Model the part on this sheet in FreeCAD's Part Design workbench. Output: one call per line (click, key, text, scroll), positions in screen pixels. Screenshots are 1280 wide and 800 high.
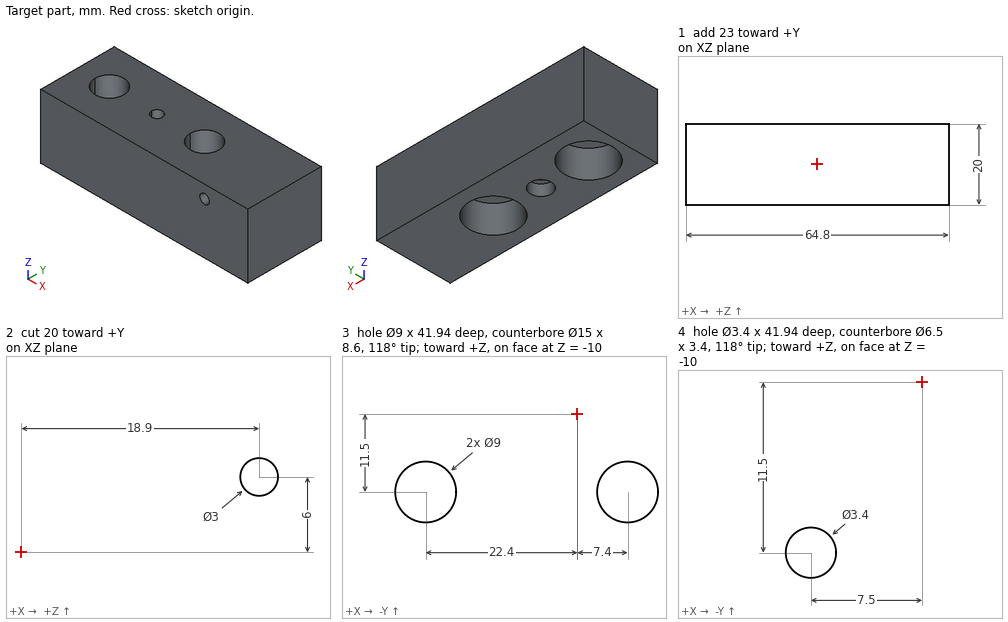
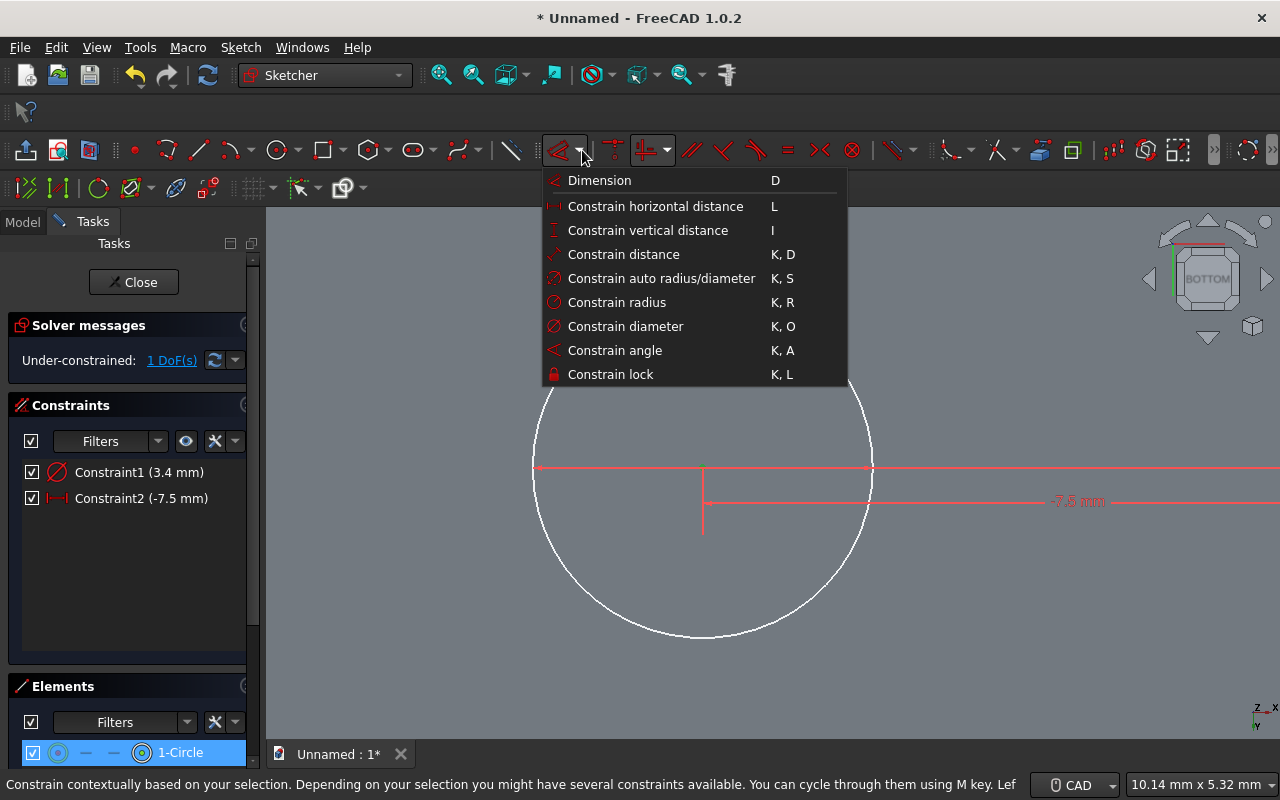
click(695, 230)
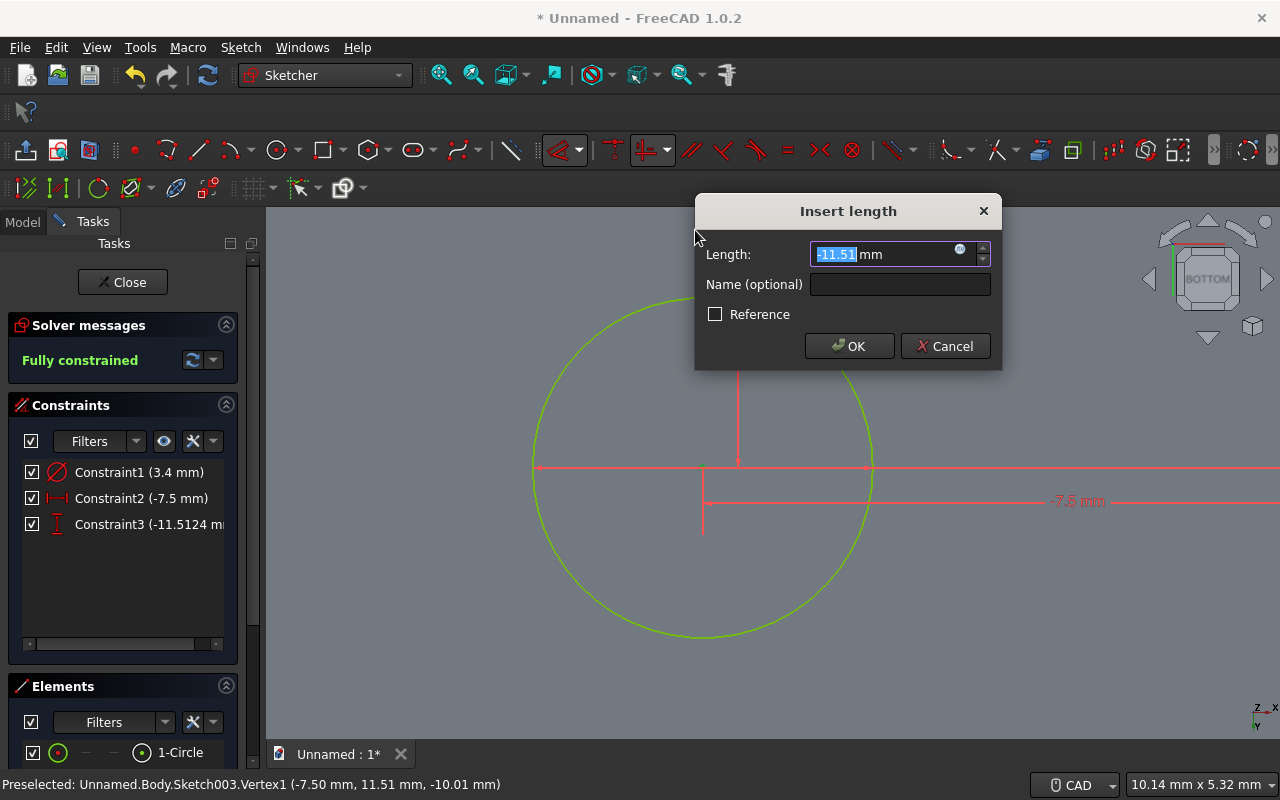
text(-11.5)
key(Return)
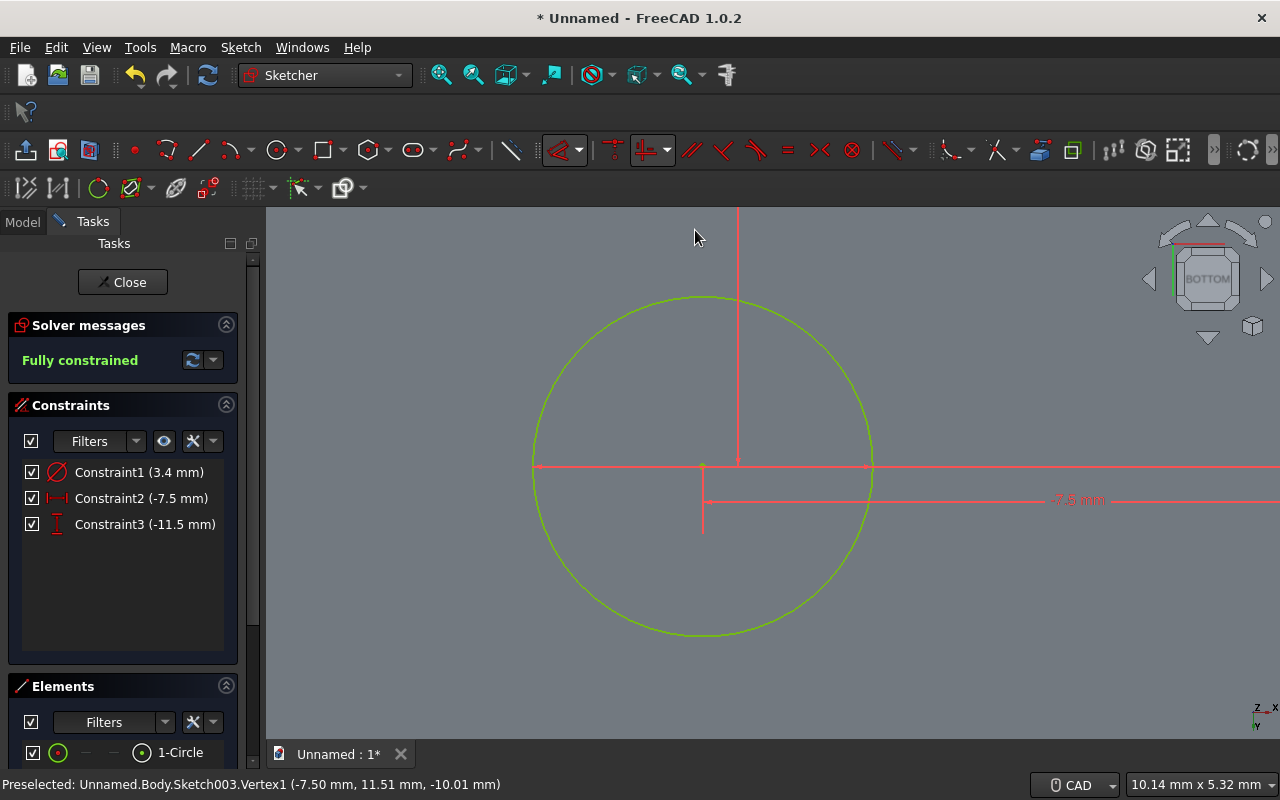
click(123, 282)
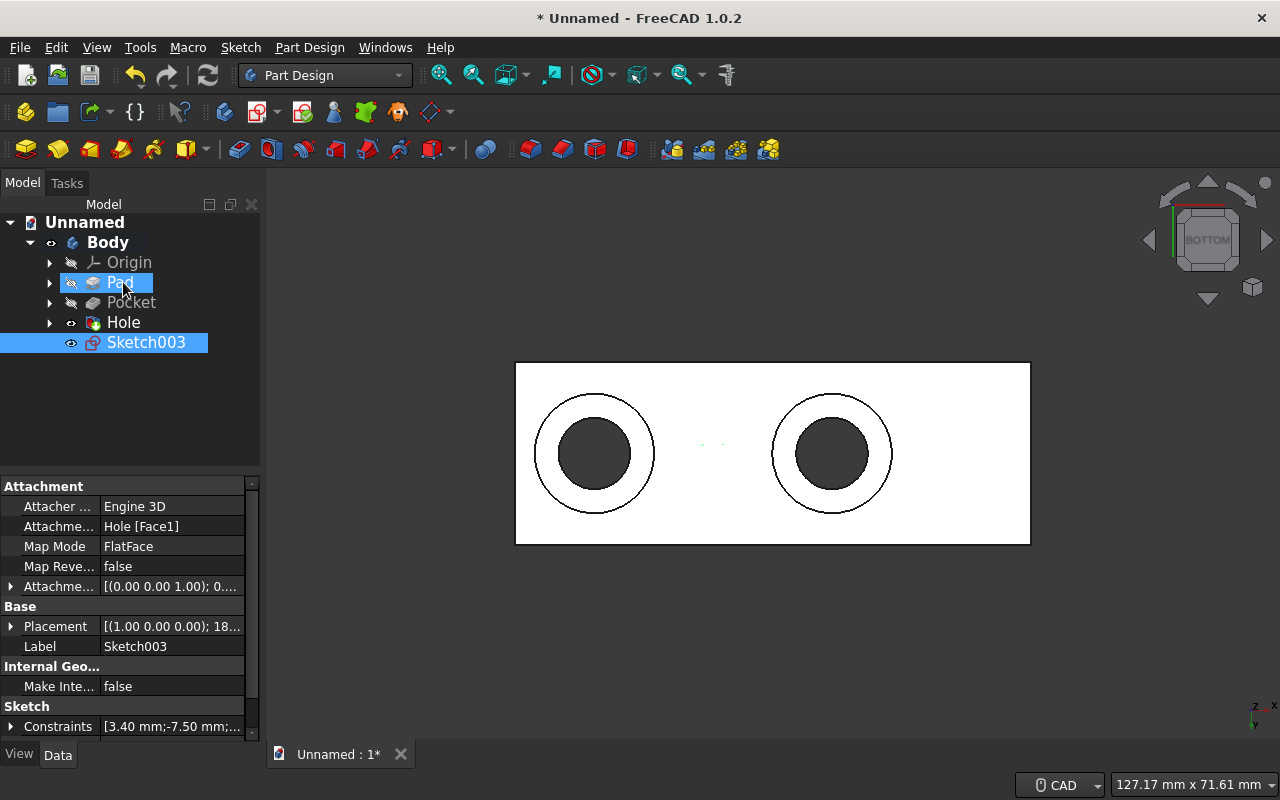
click(272, 150)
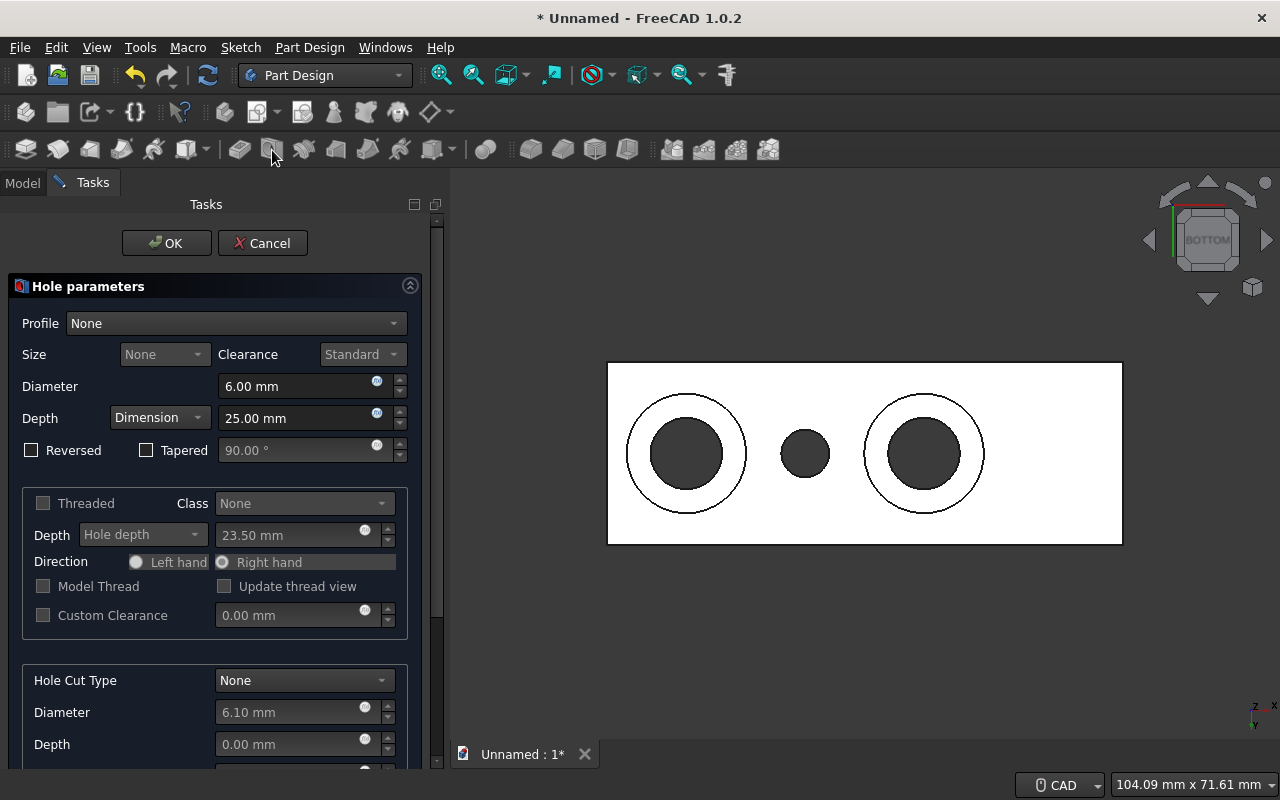
triple_click(305, 386)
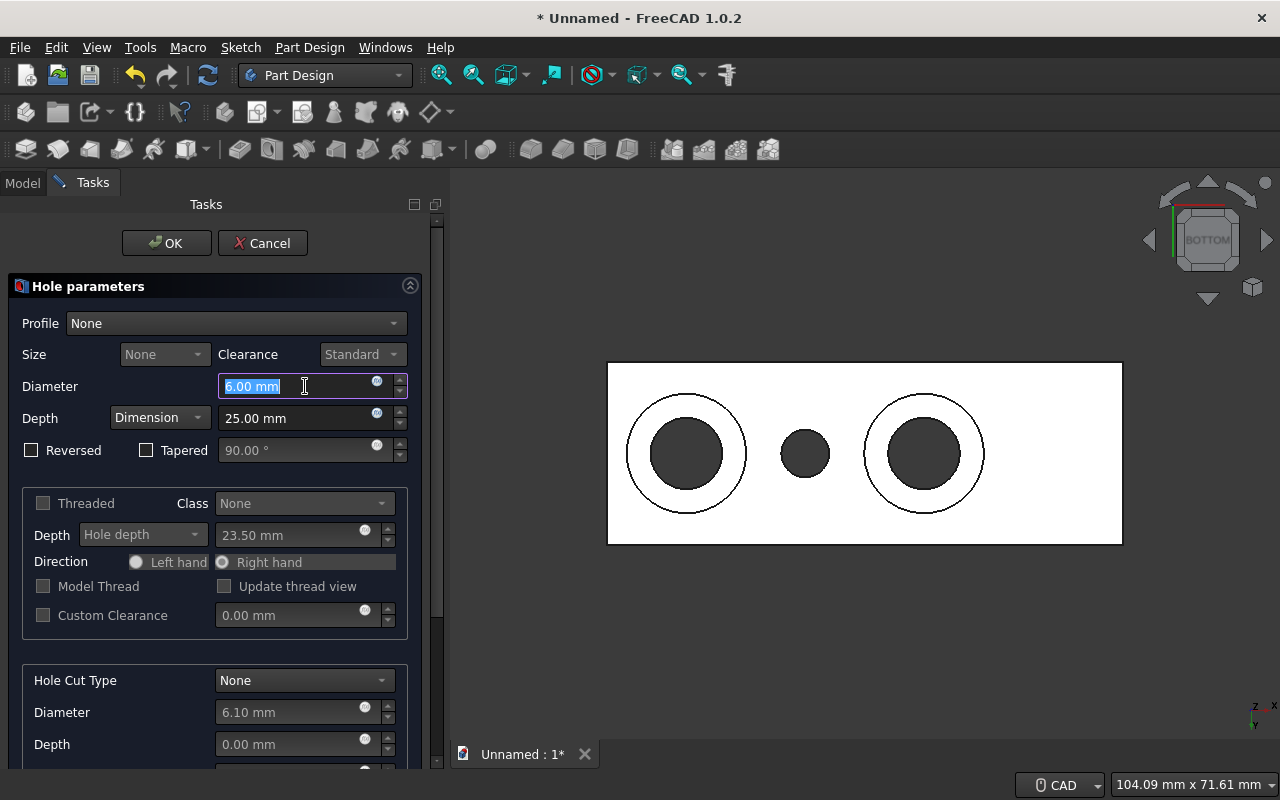
text(3.4)
key(Tab)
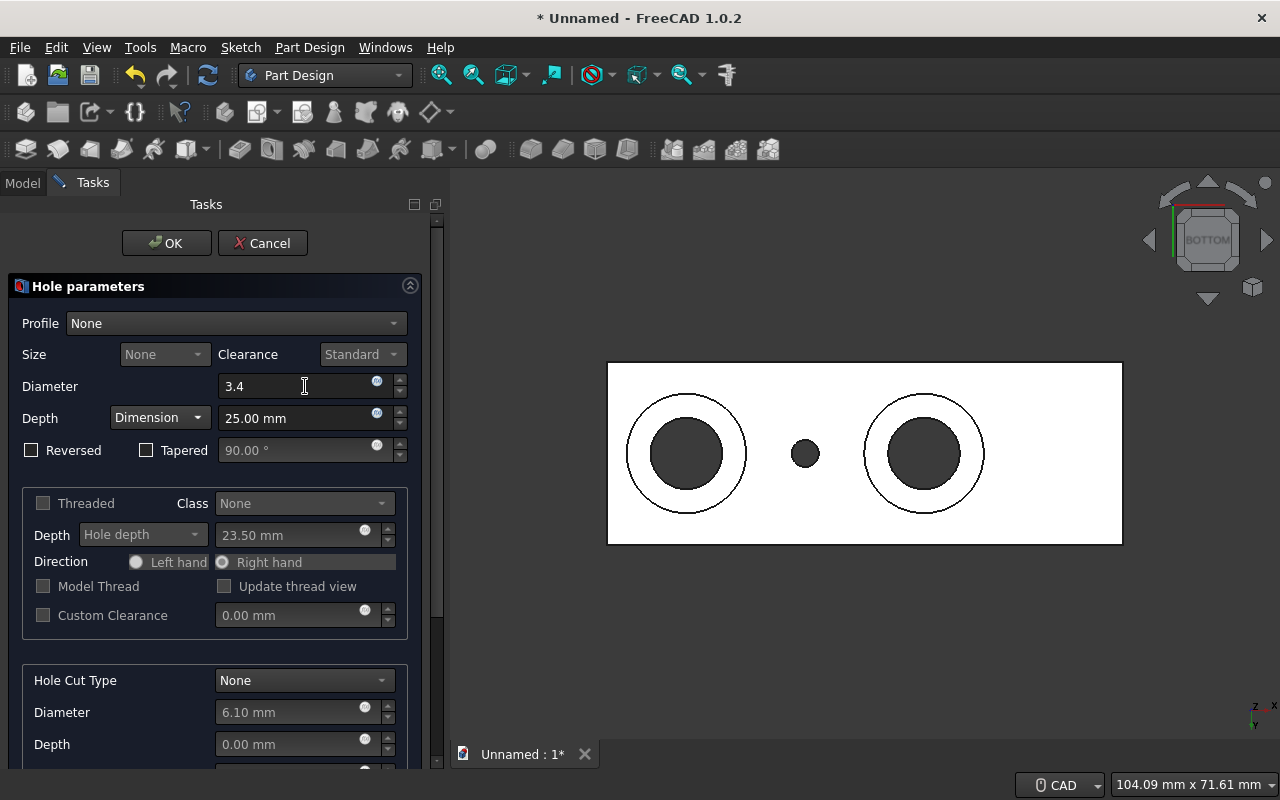
triple_click(305, 418)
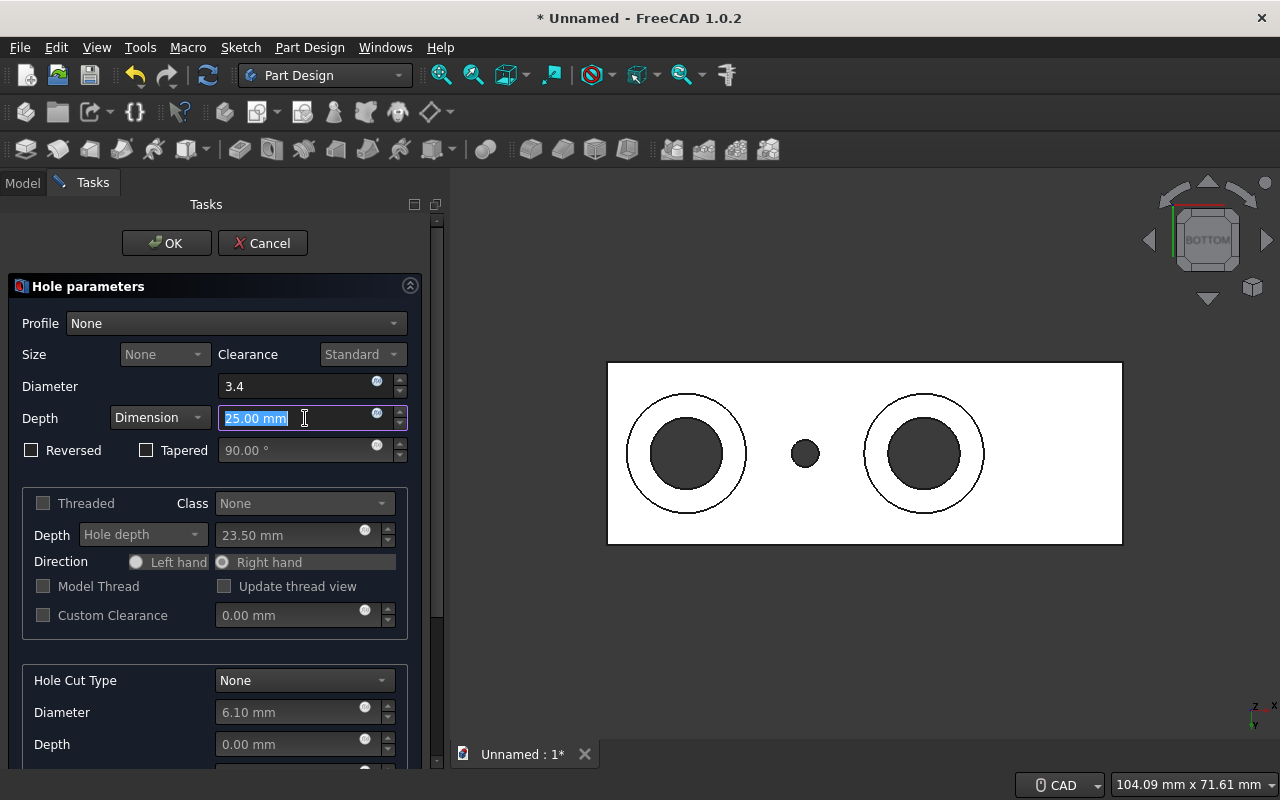
text(41.94)
key(Tab)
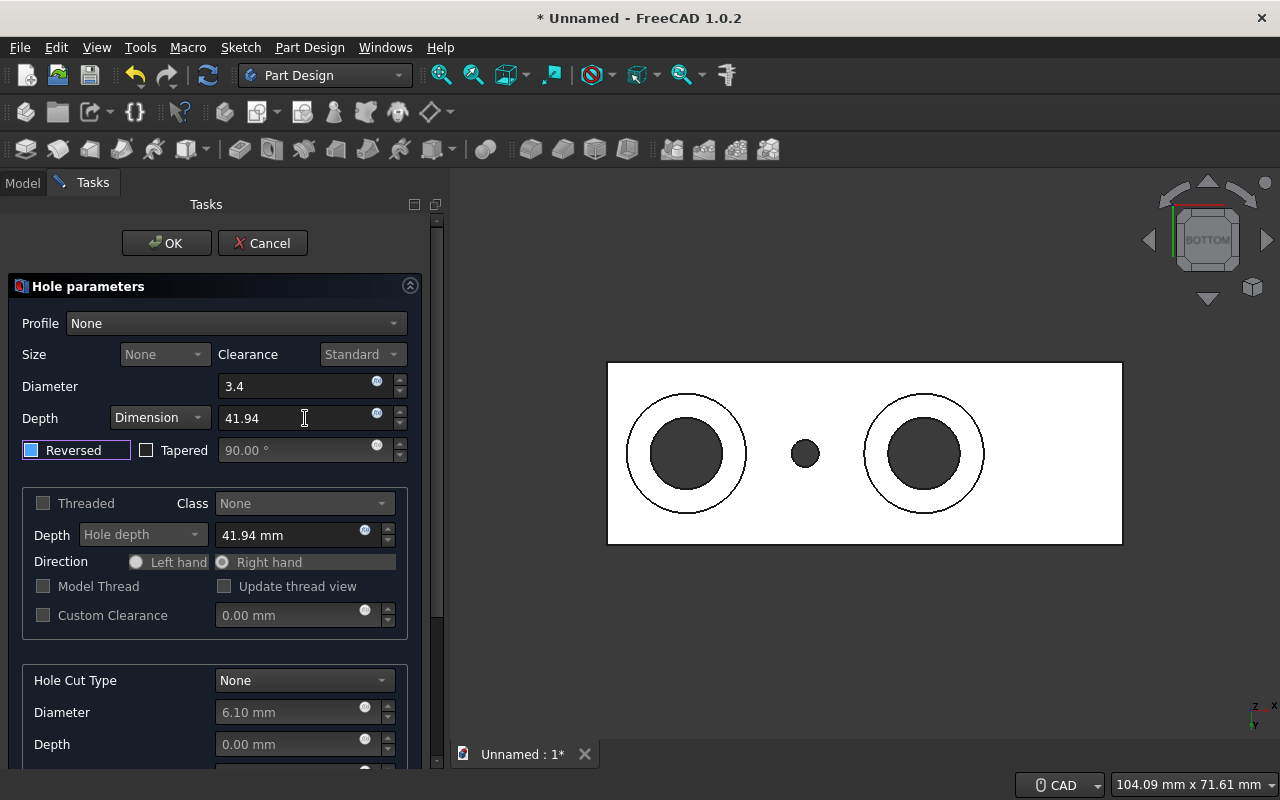
click(306, 680)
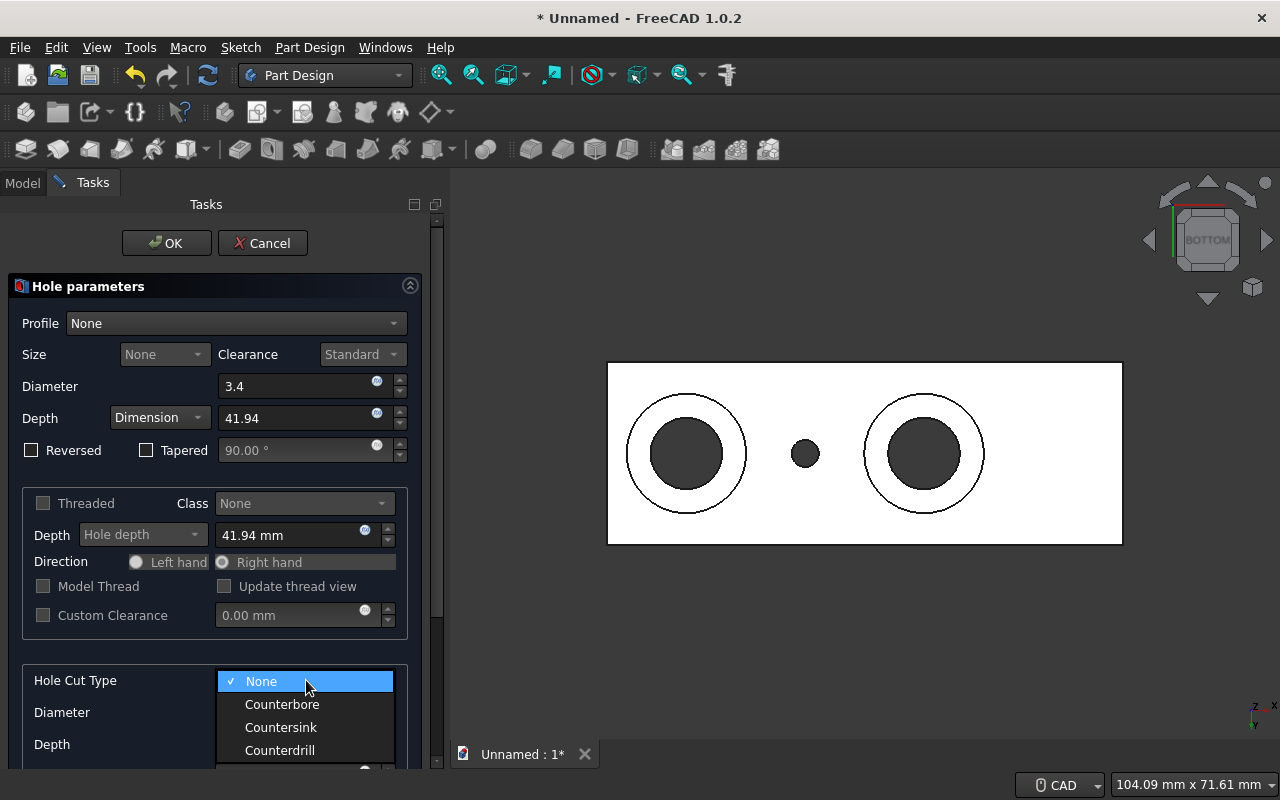
click(304, 704)